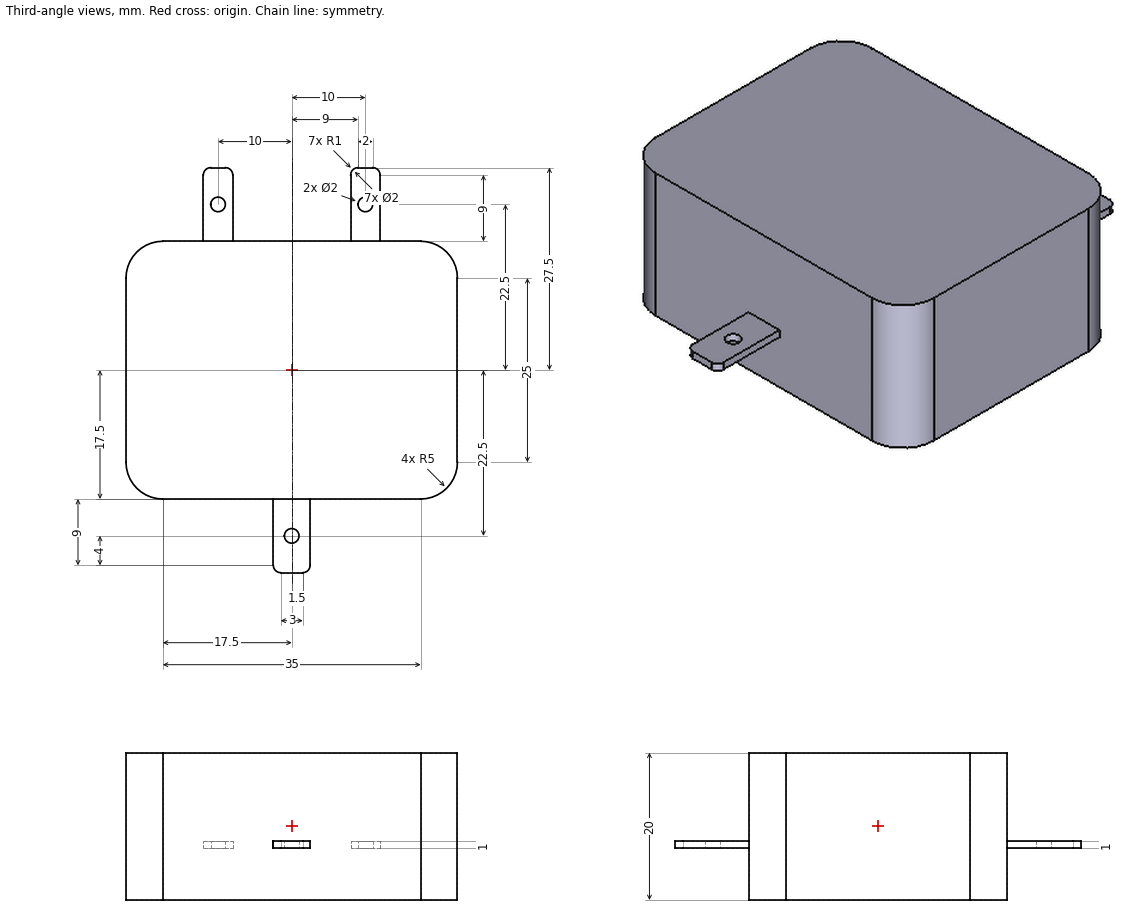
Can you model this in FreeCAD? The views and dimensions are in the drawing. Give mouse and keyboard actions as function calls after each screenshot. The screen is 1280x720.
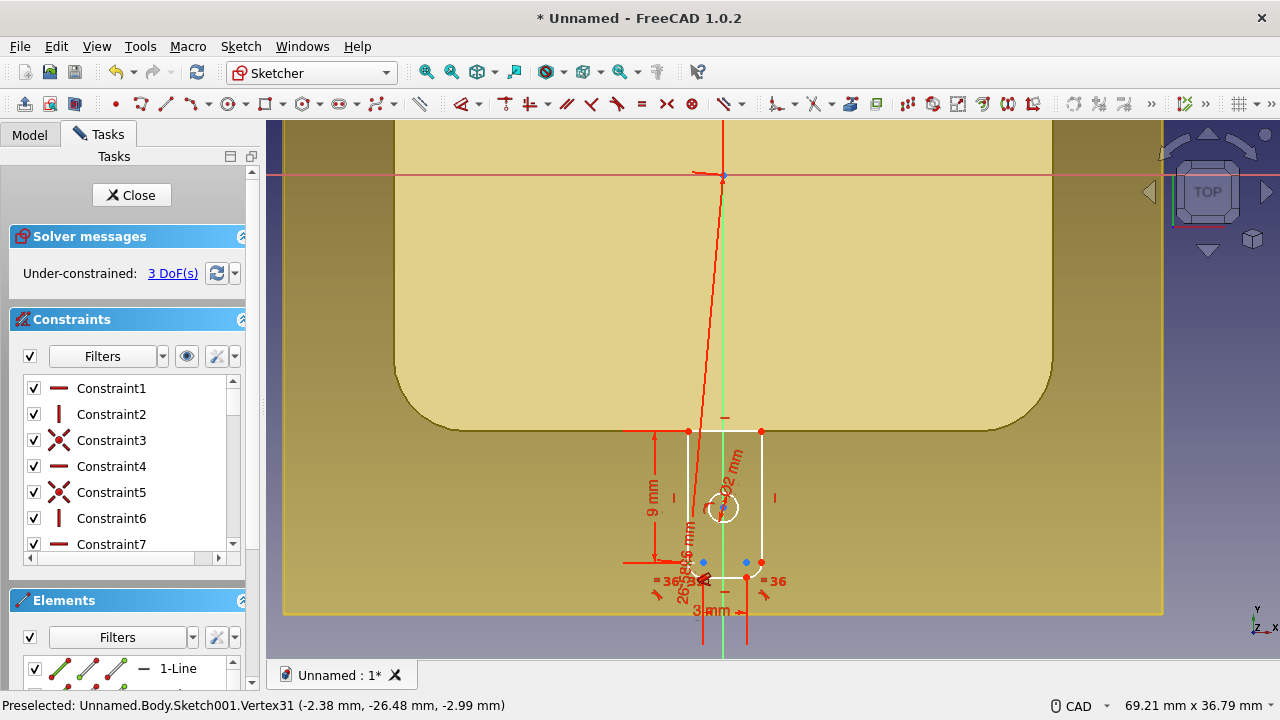
click(723, 508)
click(654, 535)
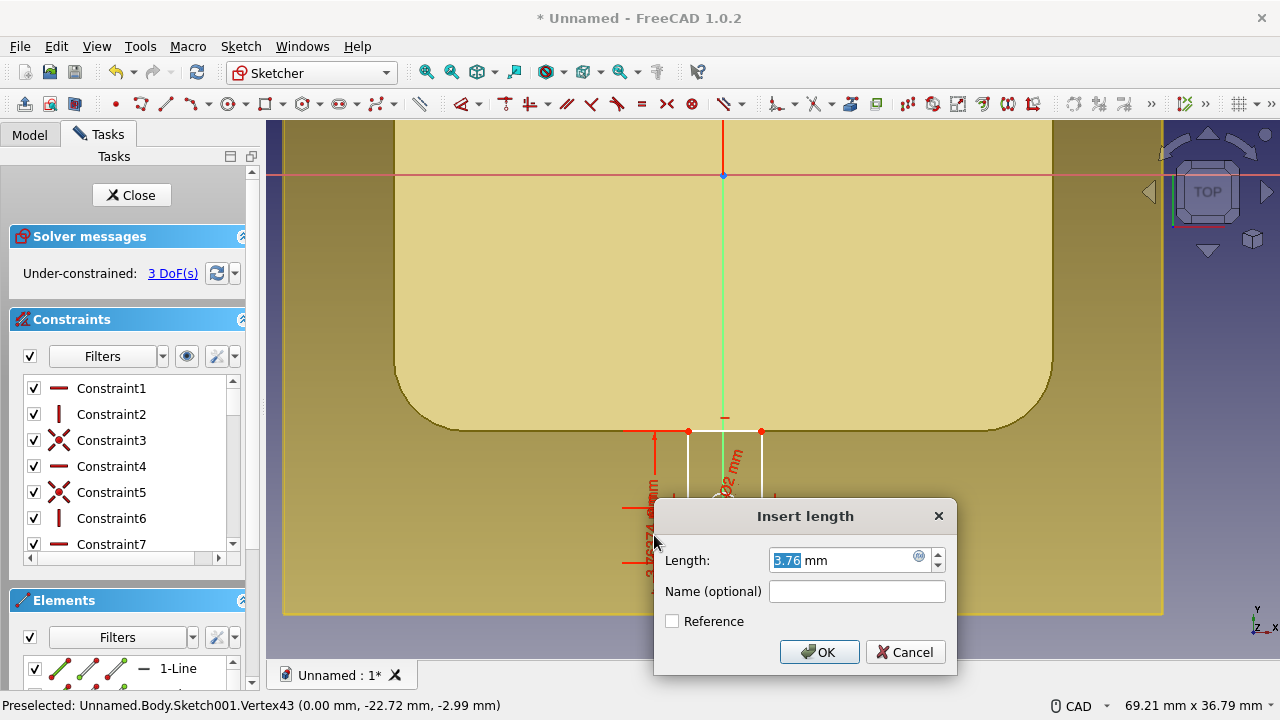
text(4)
key(Return)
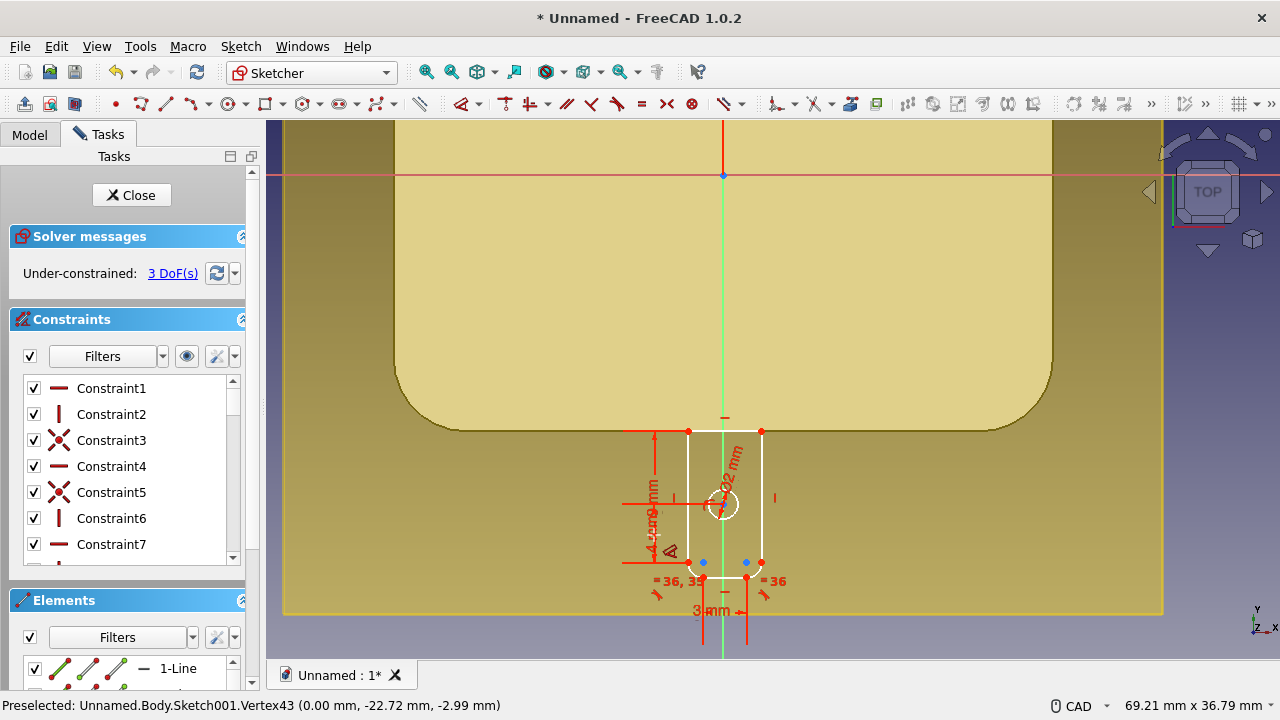
scroll(747, 578, up, 3)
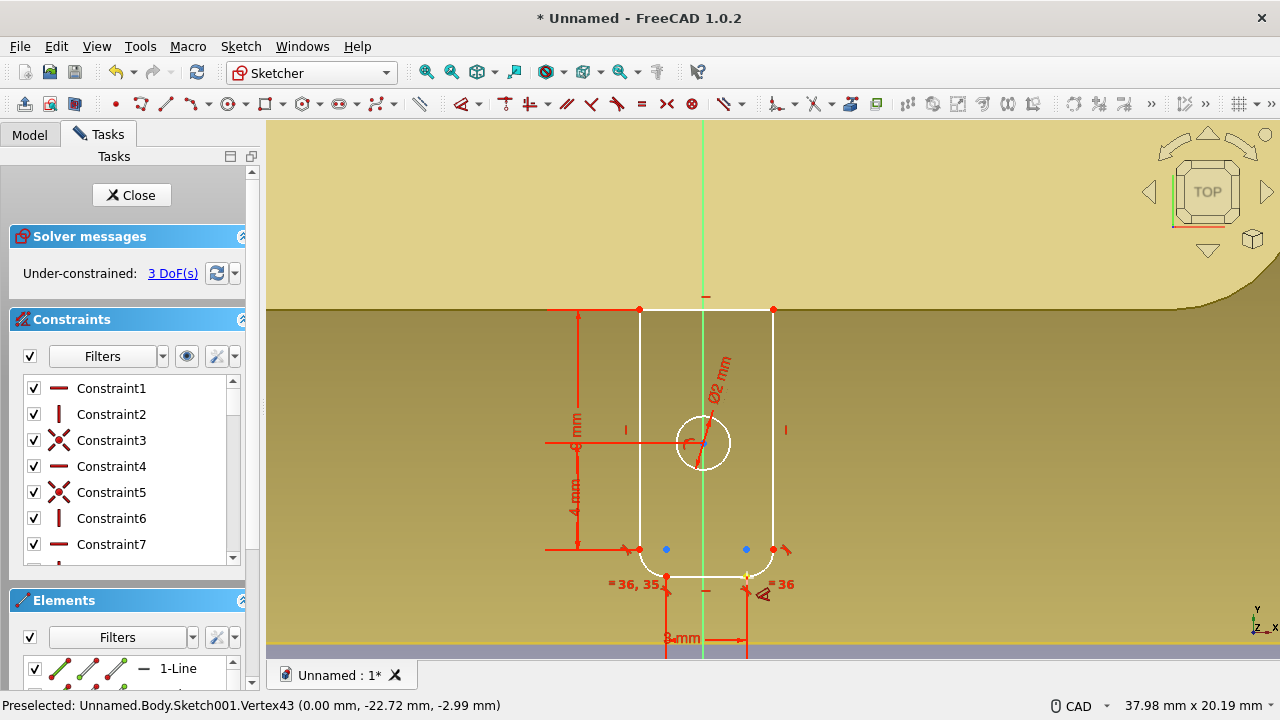
click(747, 577)
click(725, 611)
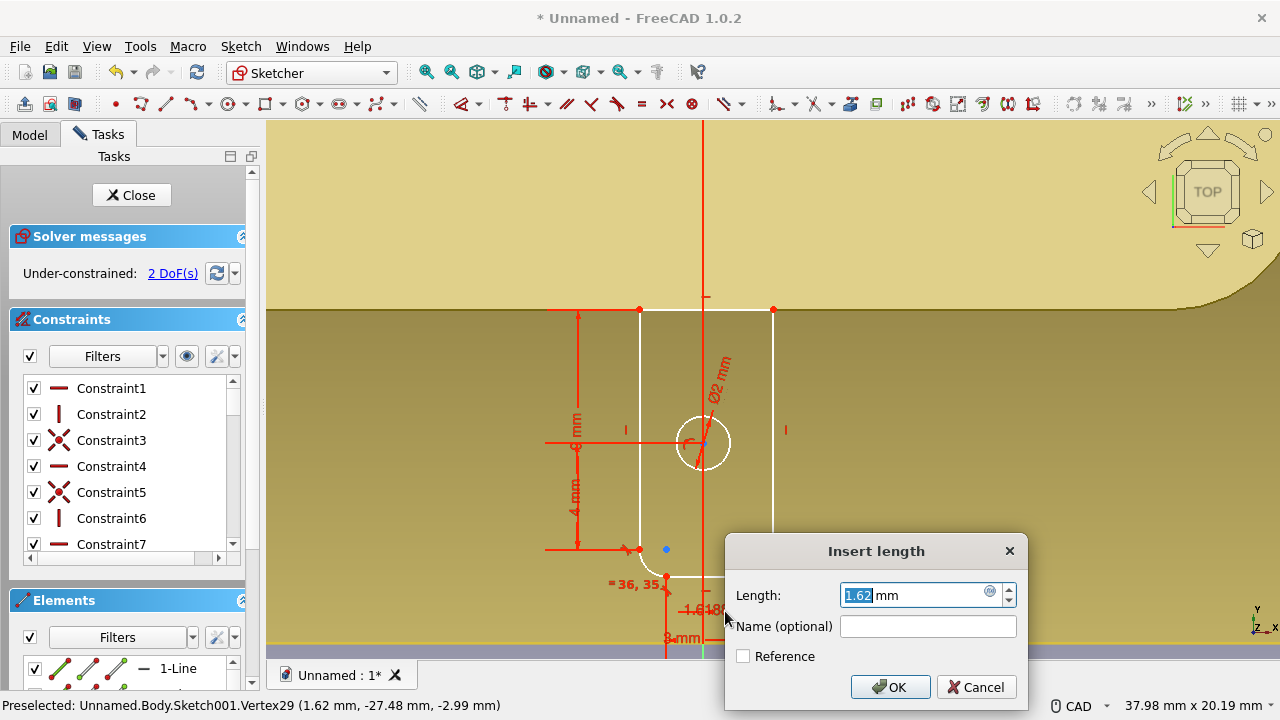
text(1.5)
key(Return)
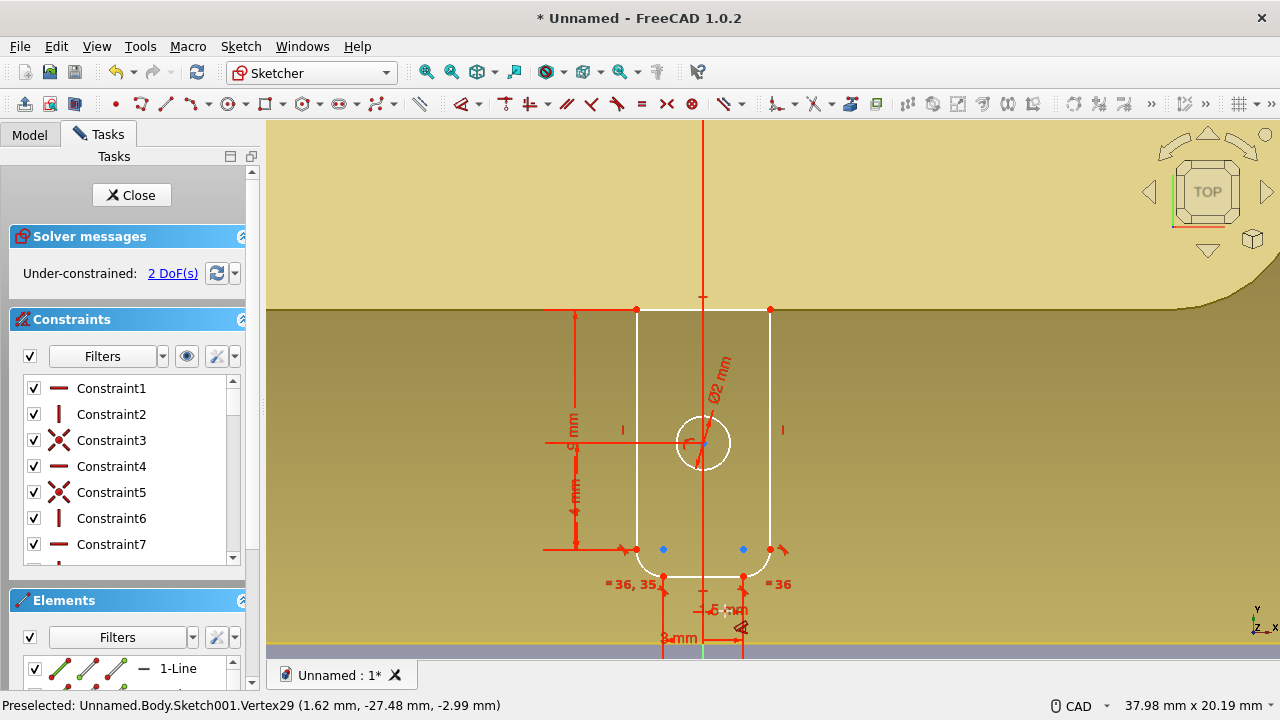
scroll(705, 568, down, 7)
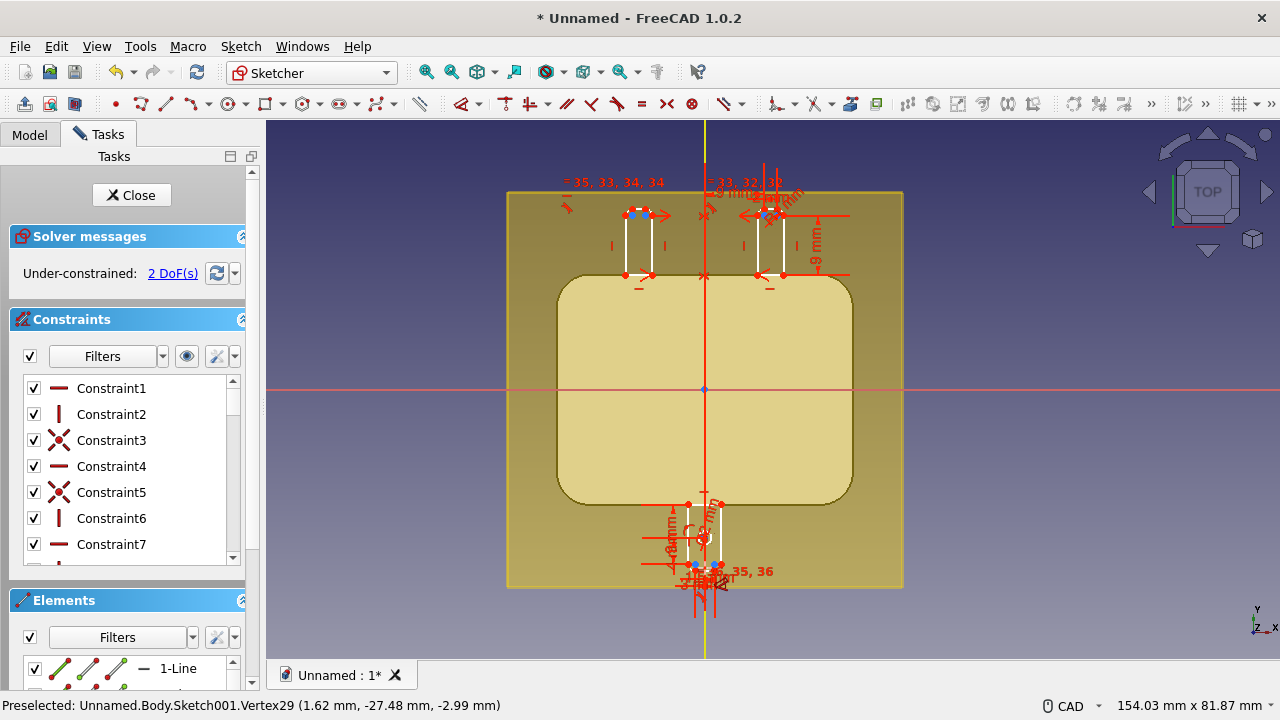
click(705, 538)
click(739, 464)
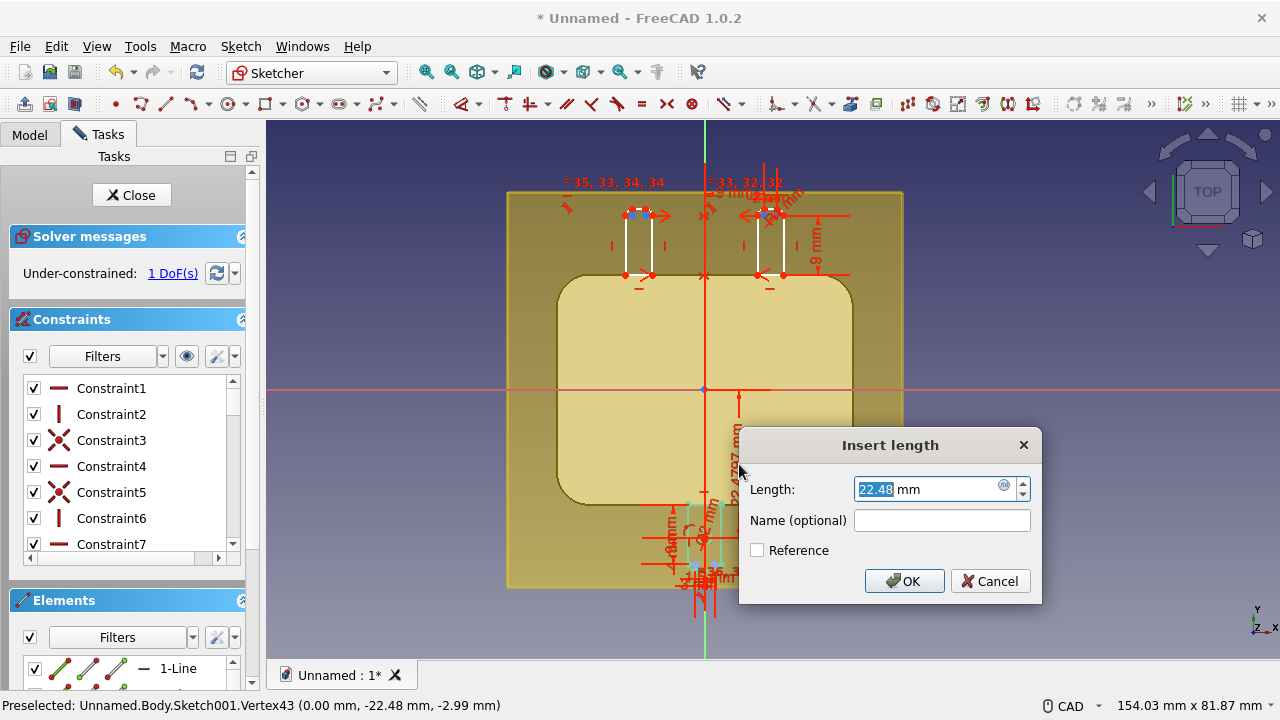
text(22.5)
key(Return)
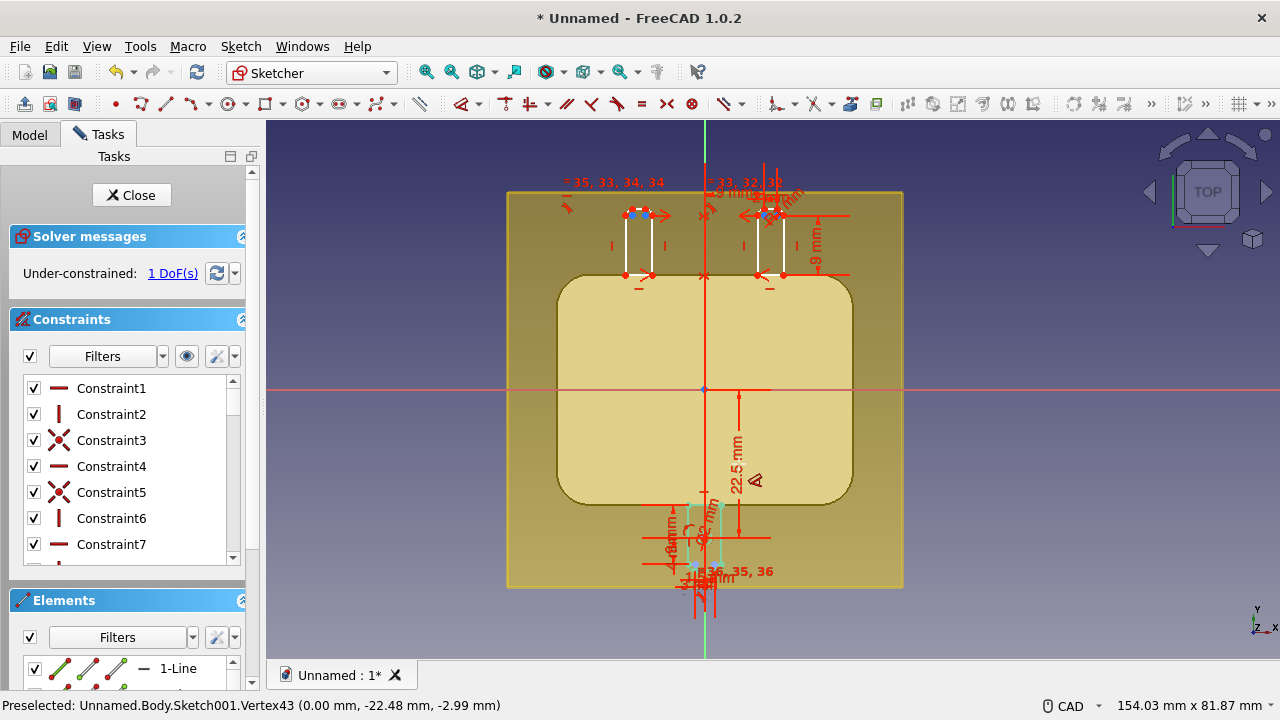
scroll(764, 209, up, 4)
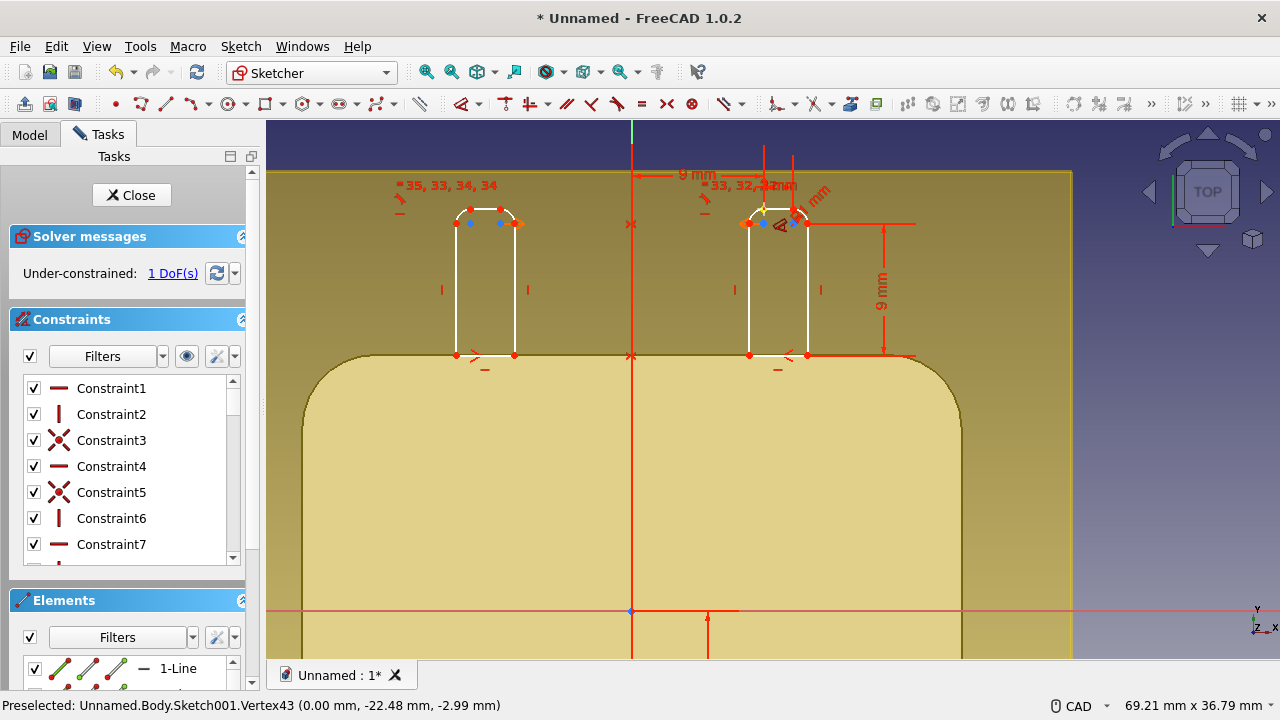
click(764, 209)
click(798, 410)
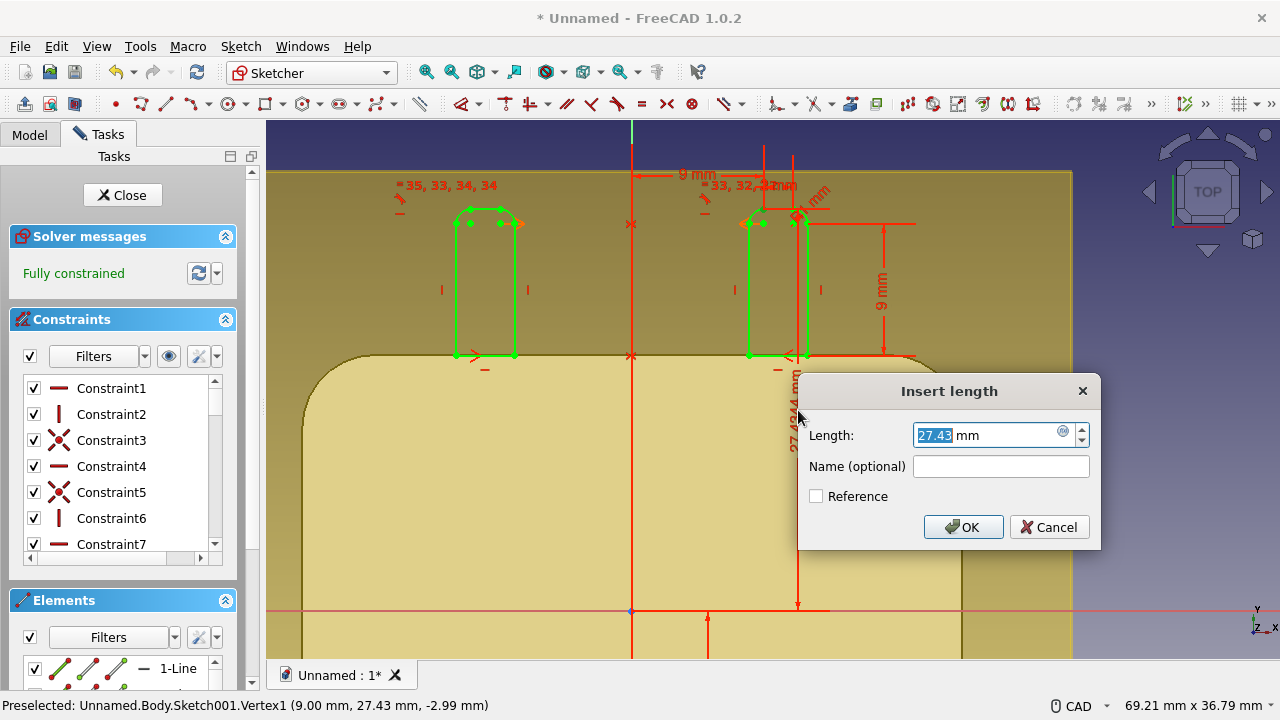
text(27.5)
key(Return)
key(Escape)